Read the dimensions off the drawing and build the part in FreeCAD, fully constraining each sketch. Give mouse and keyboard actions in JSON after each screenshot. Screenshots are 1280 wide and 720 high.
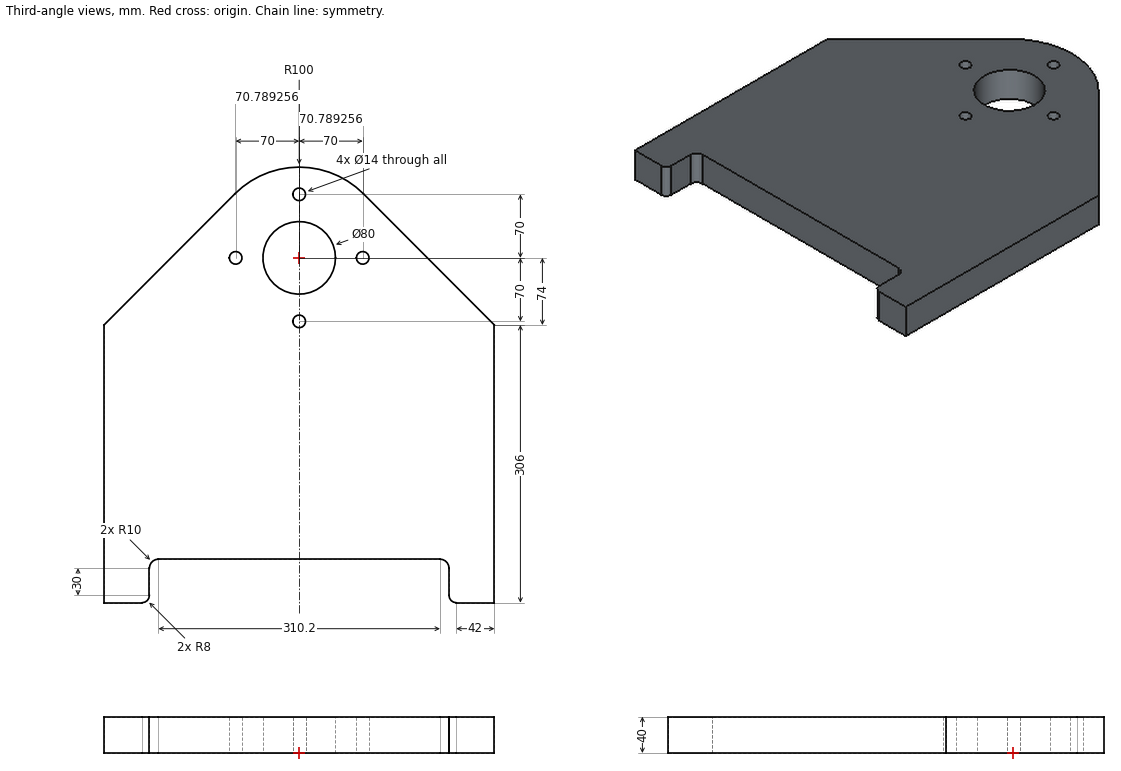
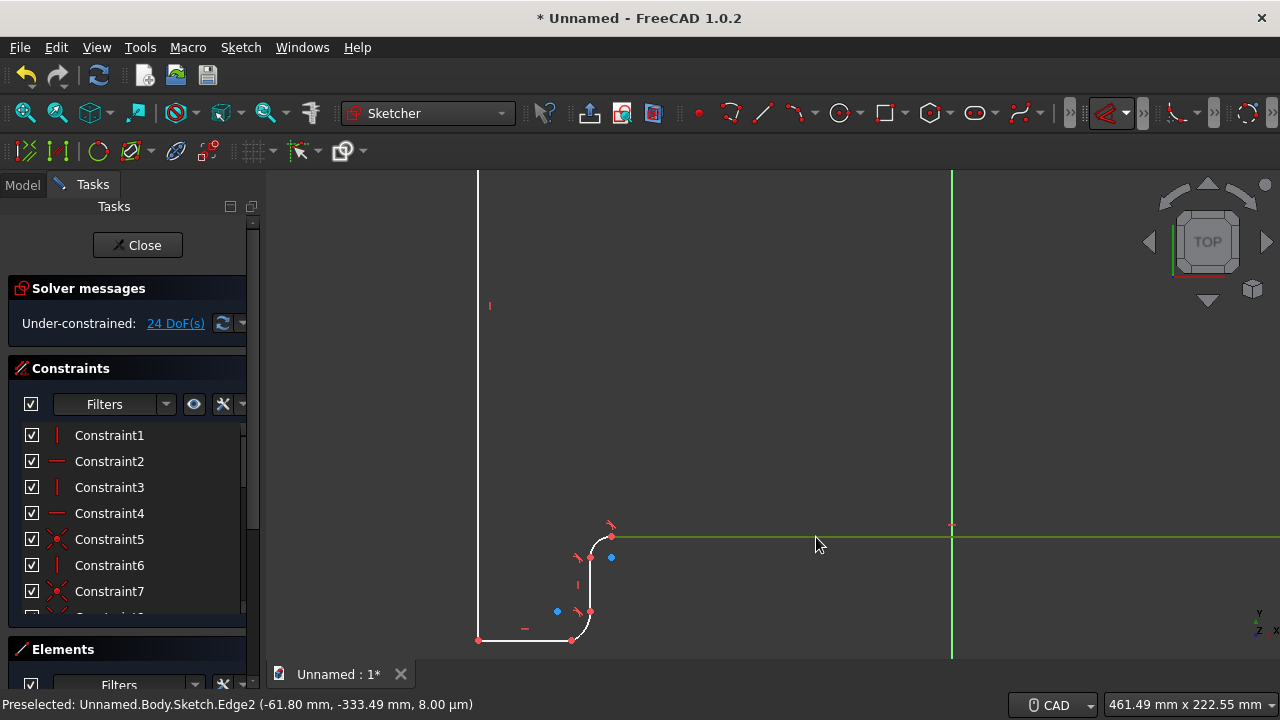
{"action": "scroll", "coordinate": [598, 545], "scroll_direction": "down", "scroll_amount": 6}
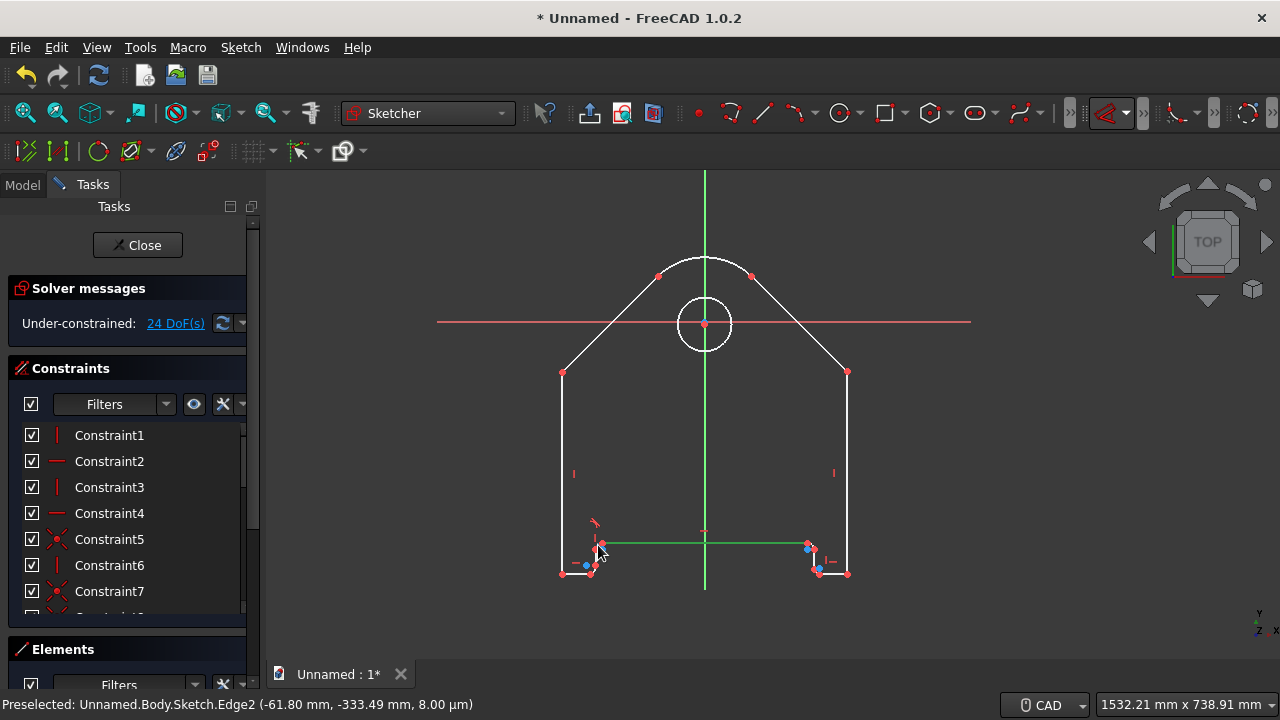
{"action": "scroll", "coordinate": [813, 547], "scroll_direction": "up", "scroll_amount": 8}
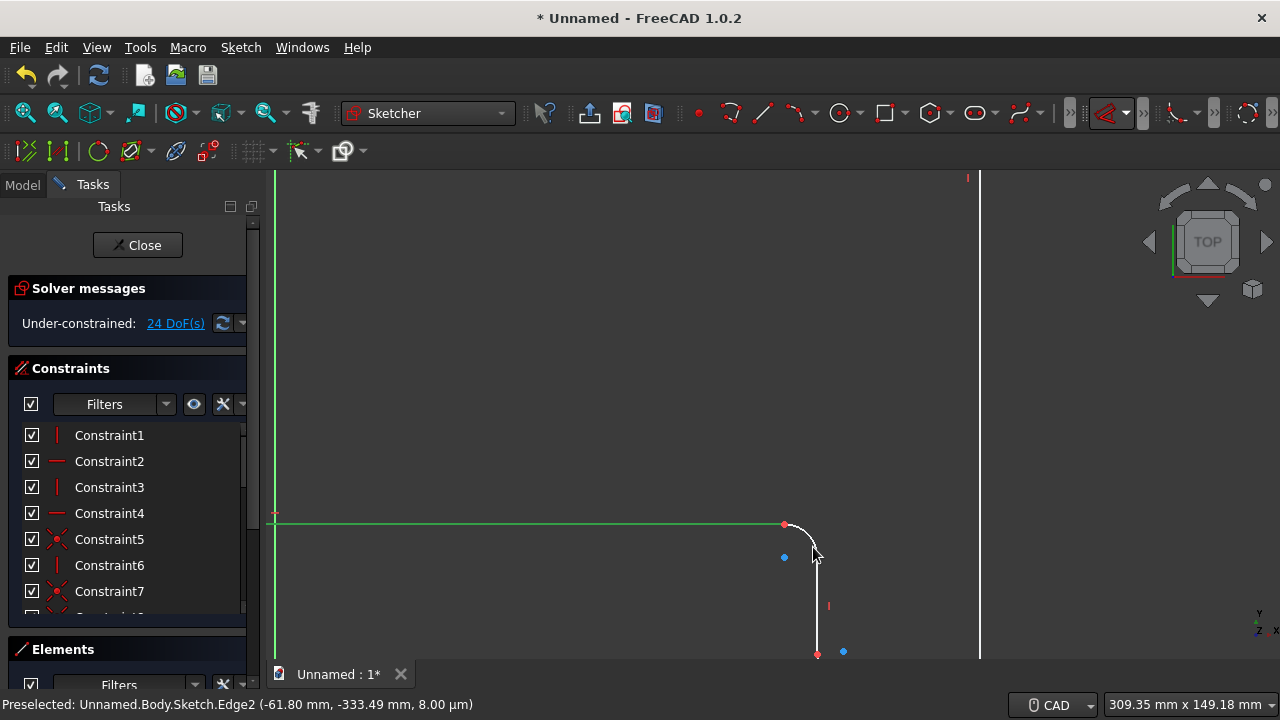
{"action": "left_click", "coordinate": [813, 542]}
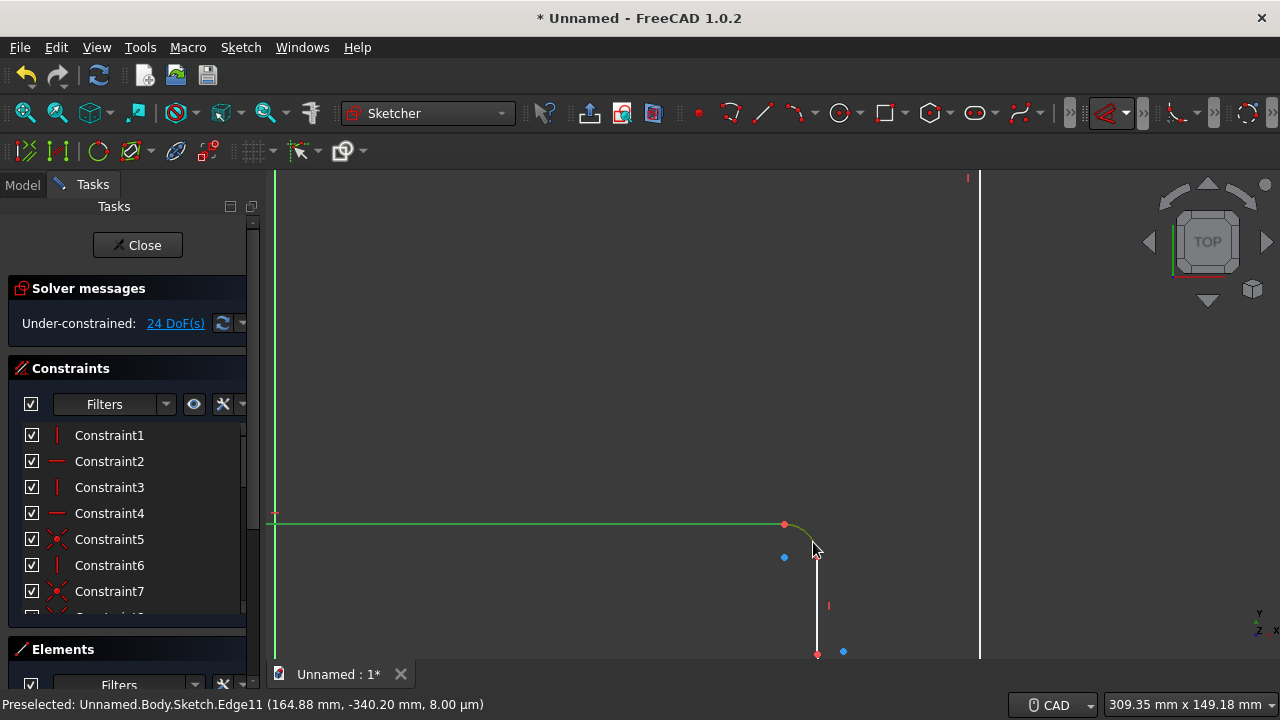
{"action": "key", "text": "t"}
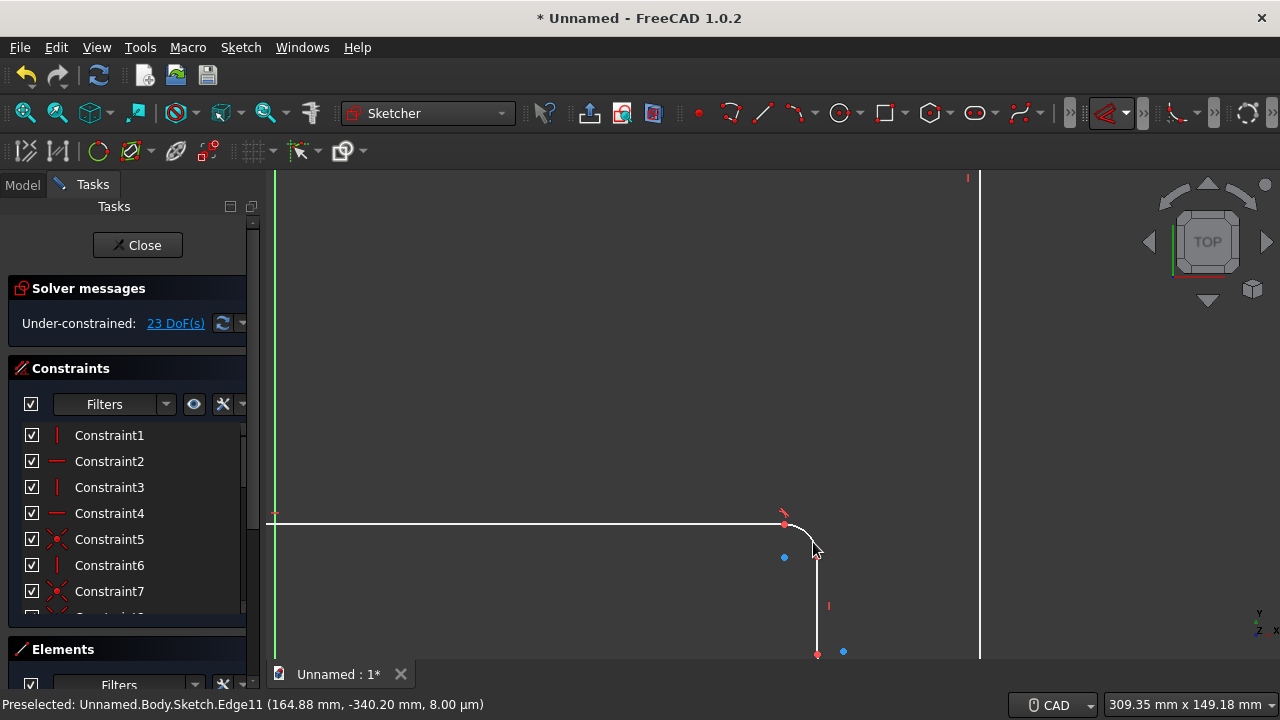
{"action": "left_click", "coordinate": [817, 586]}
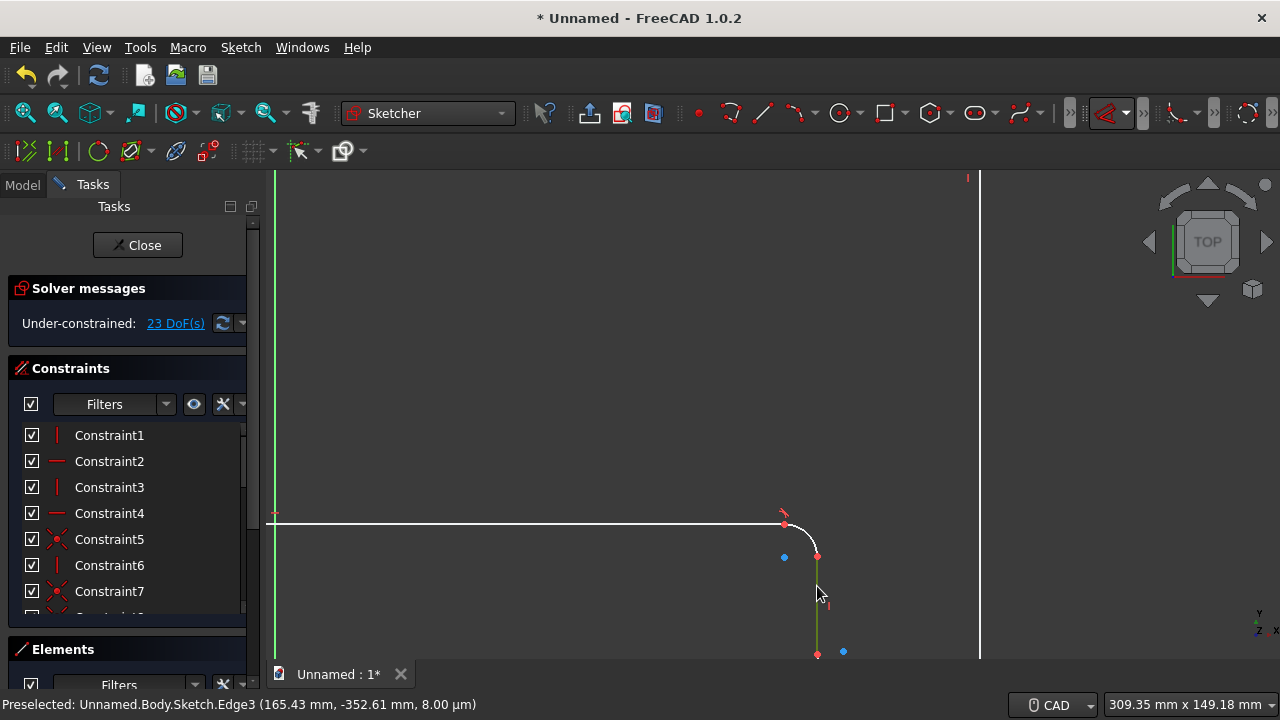
{"action": "left_click", "coordinate": [813, 542]}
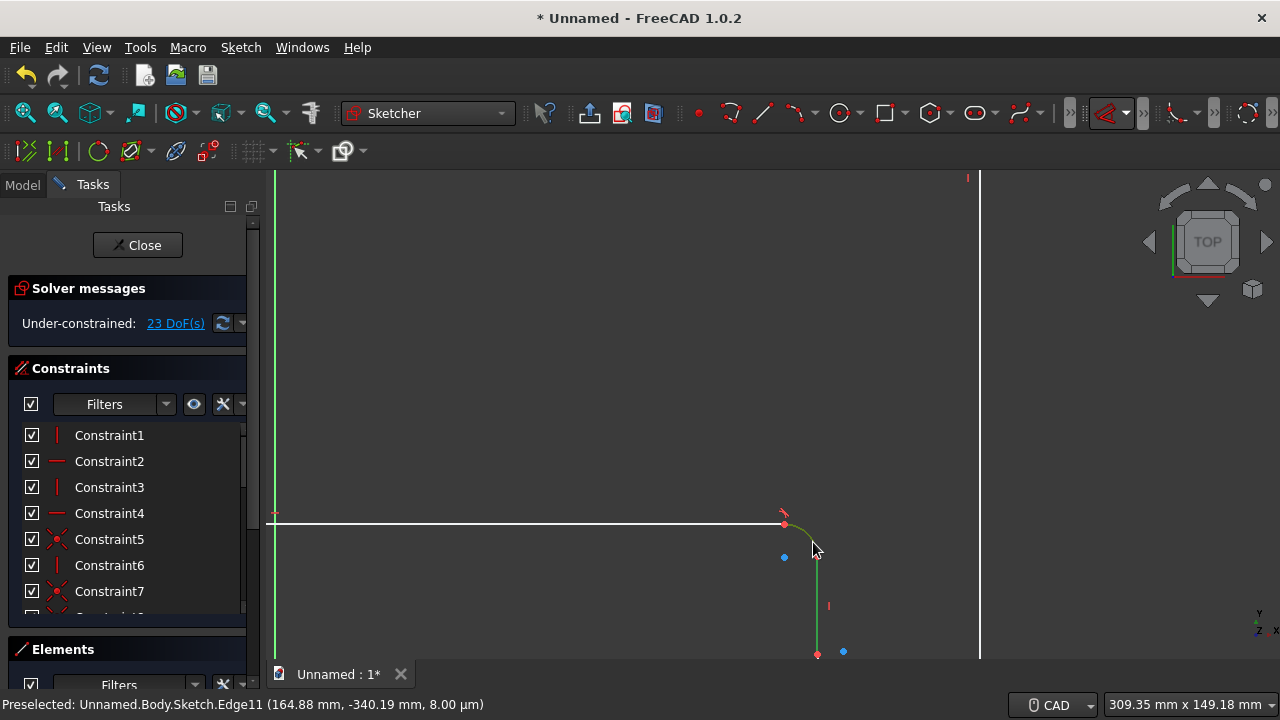
{"action": "key", "text": "t"}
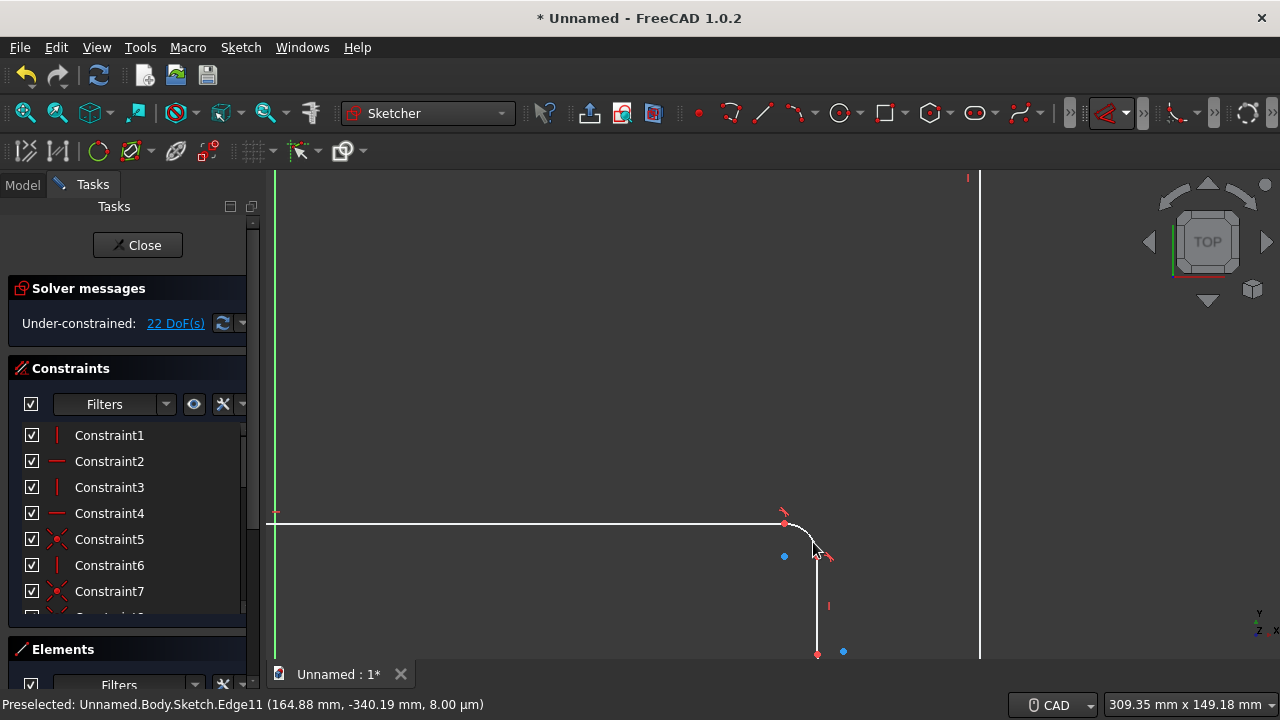
{"action": "left_click", "coordinate": [817, 586]}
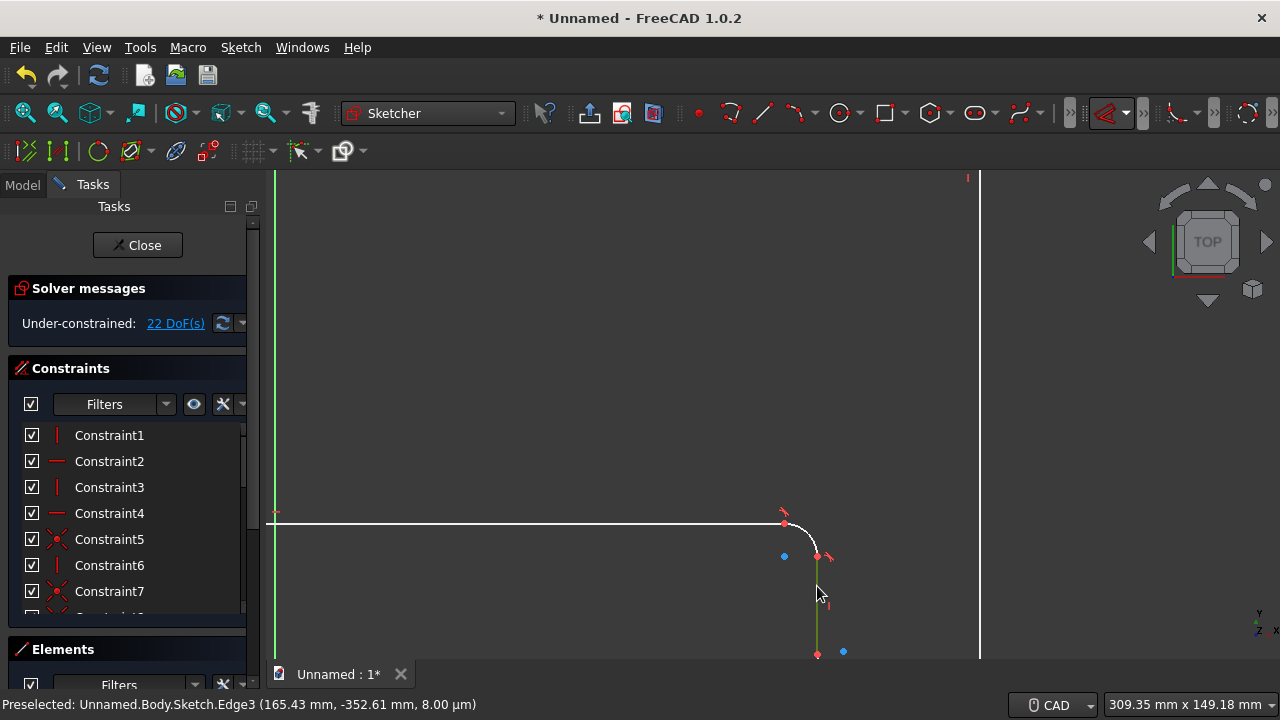
{"action": "scroll", "coordinate": [813, 547], "scroll_direction": "down", "scroll_amount": 8}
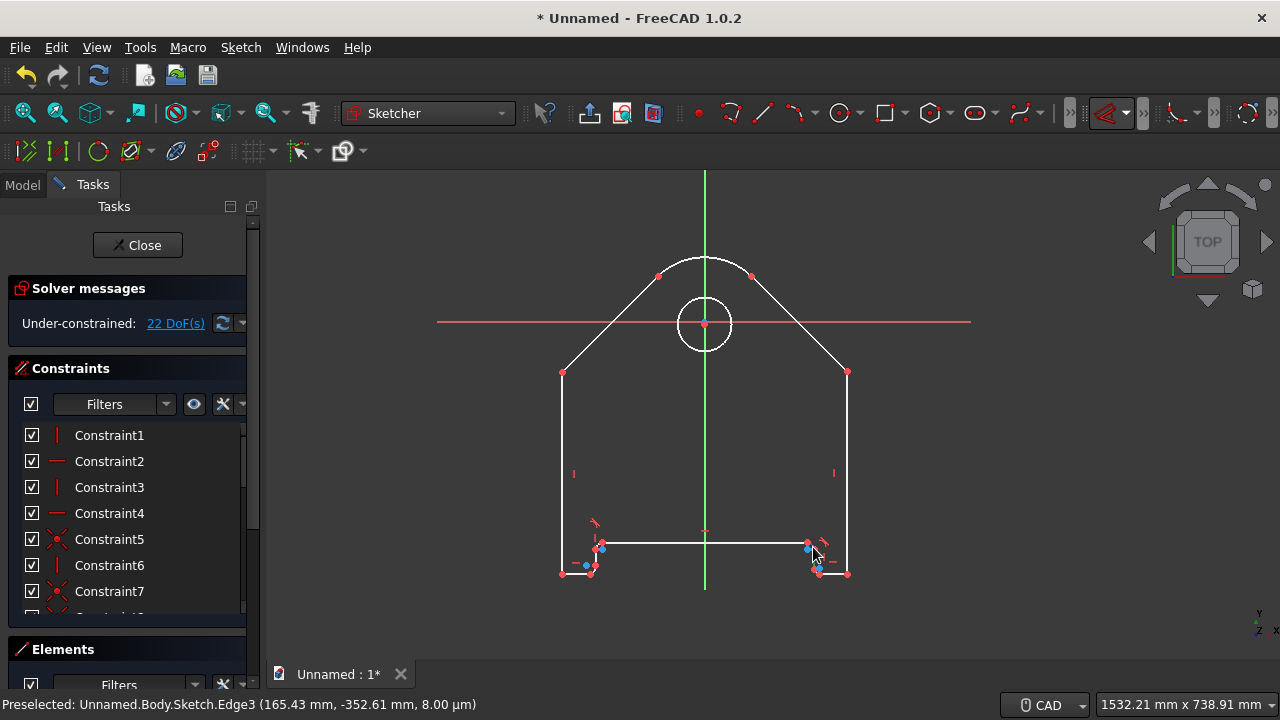
{"action": "scroll", "coordinate": [815, 571], "scroll_direction": "up", "scroll_amount": 10}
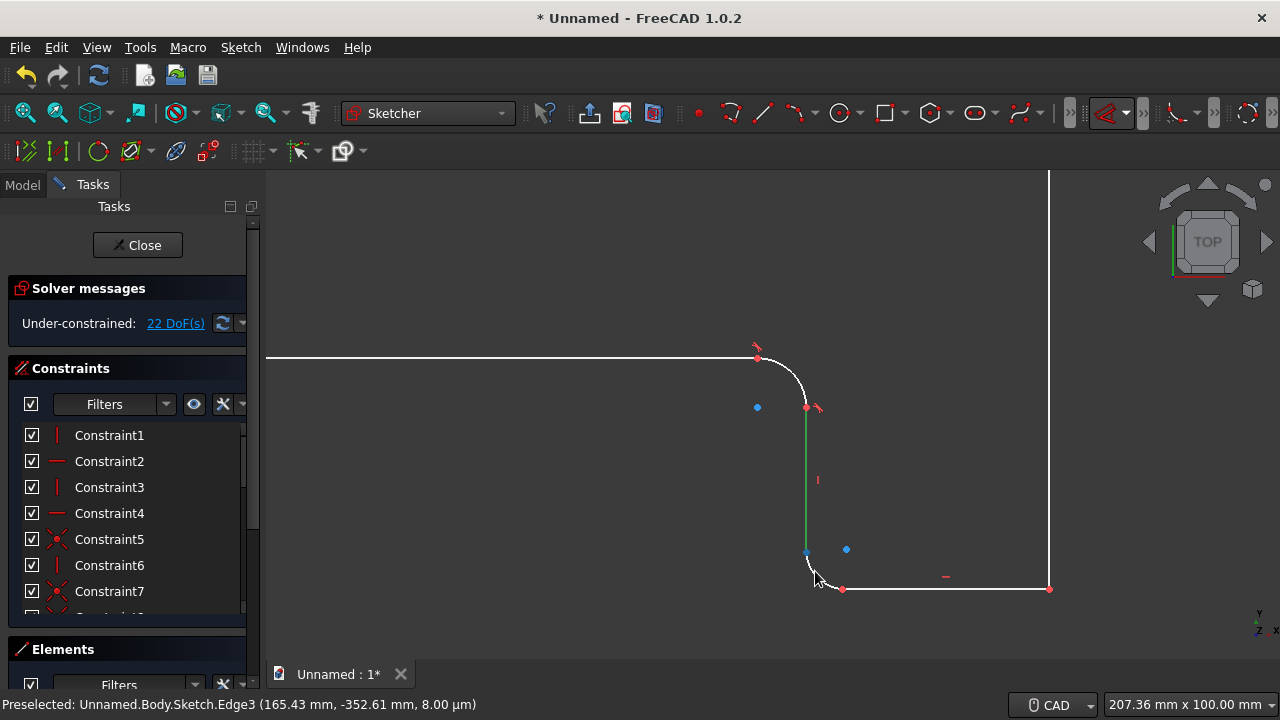
{"action": "left_click", "coordinate": [811, 569]}